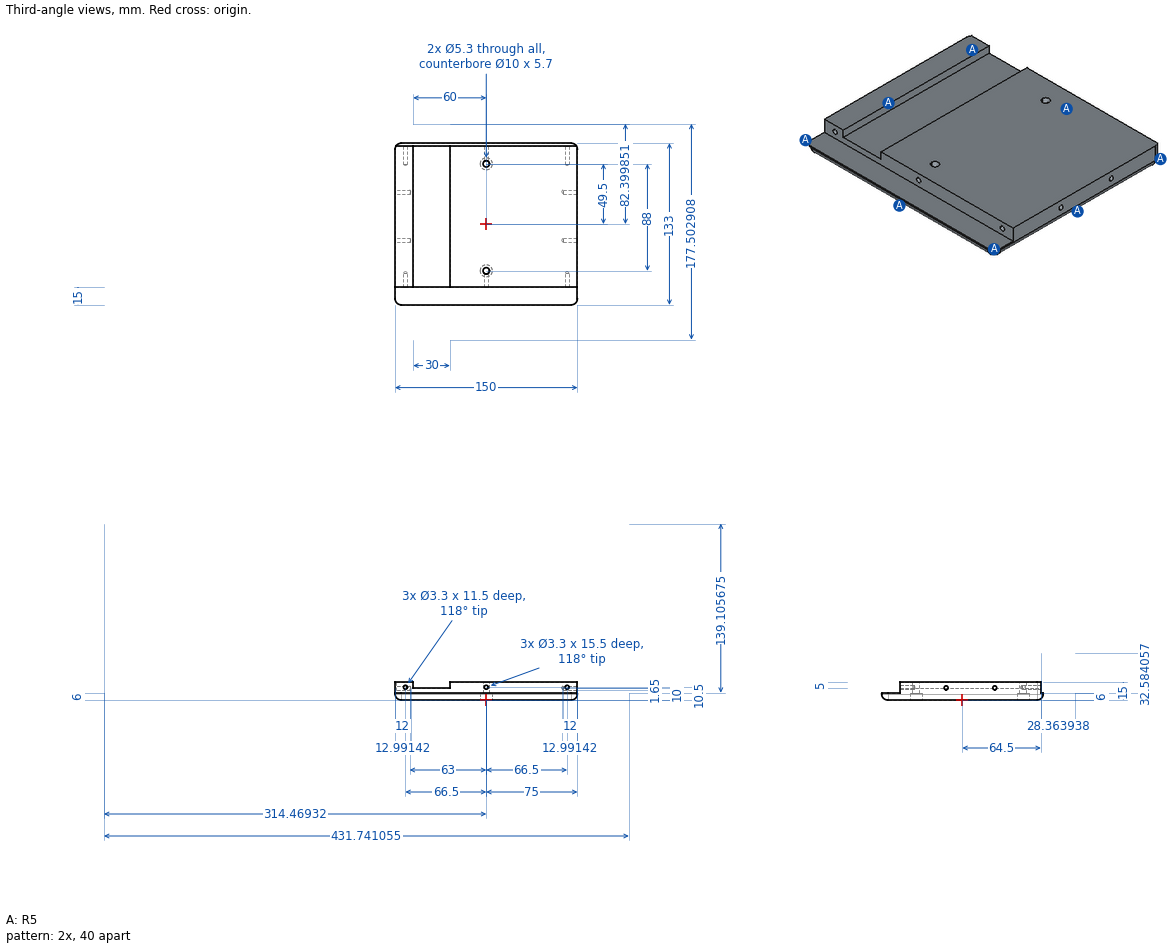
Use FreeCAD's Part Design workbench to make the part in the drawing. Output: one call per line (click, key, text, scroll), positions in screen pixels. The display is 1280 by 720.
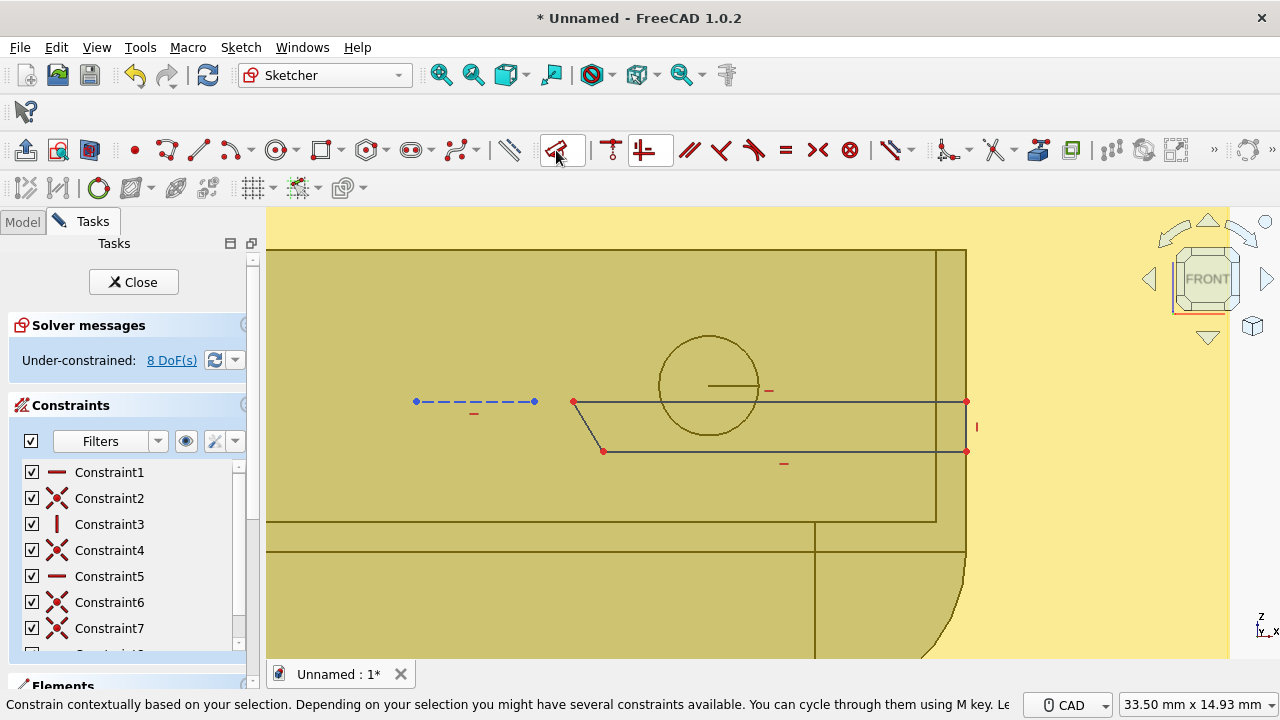
click(857, 452)
click(784, 486)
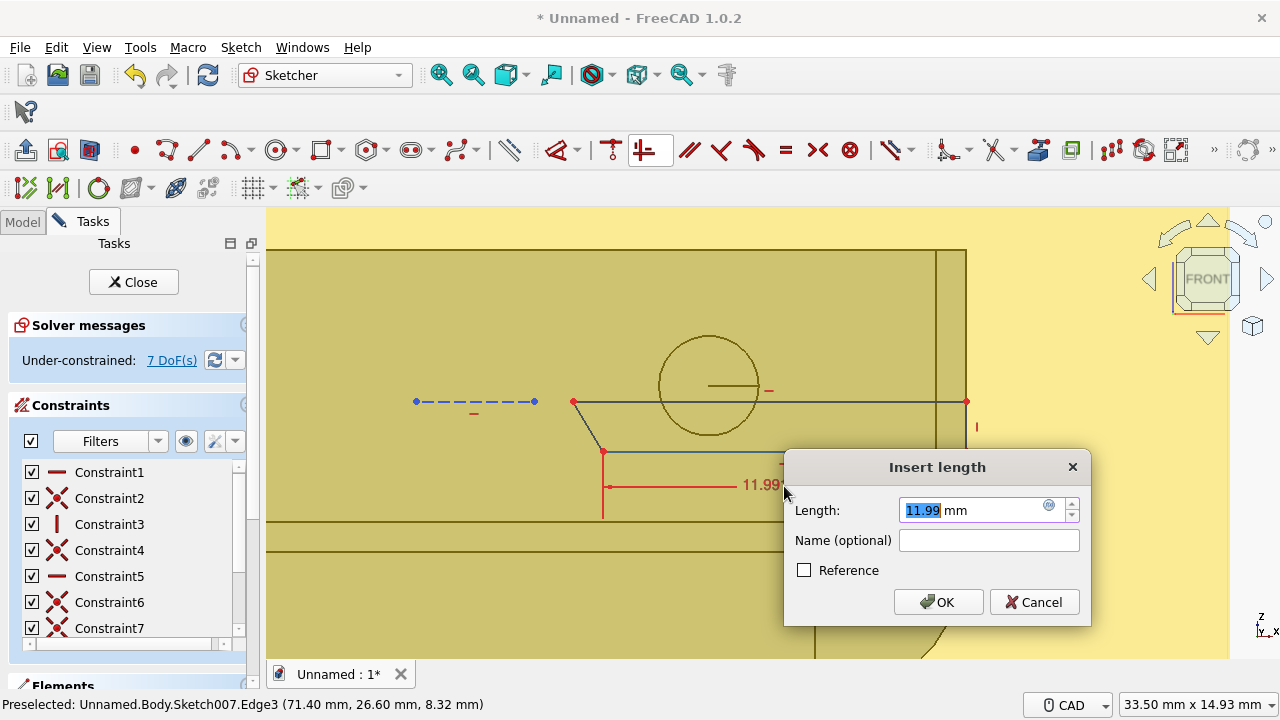
text(12)
key(Return)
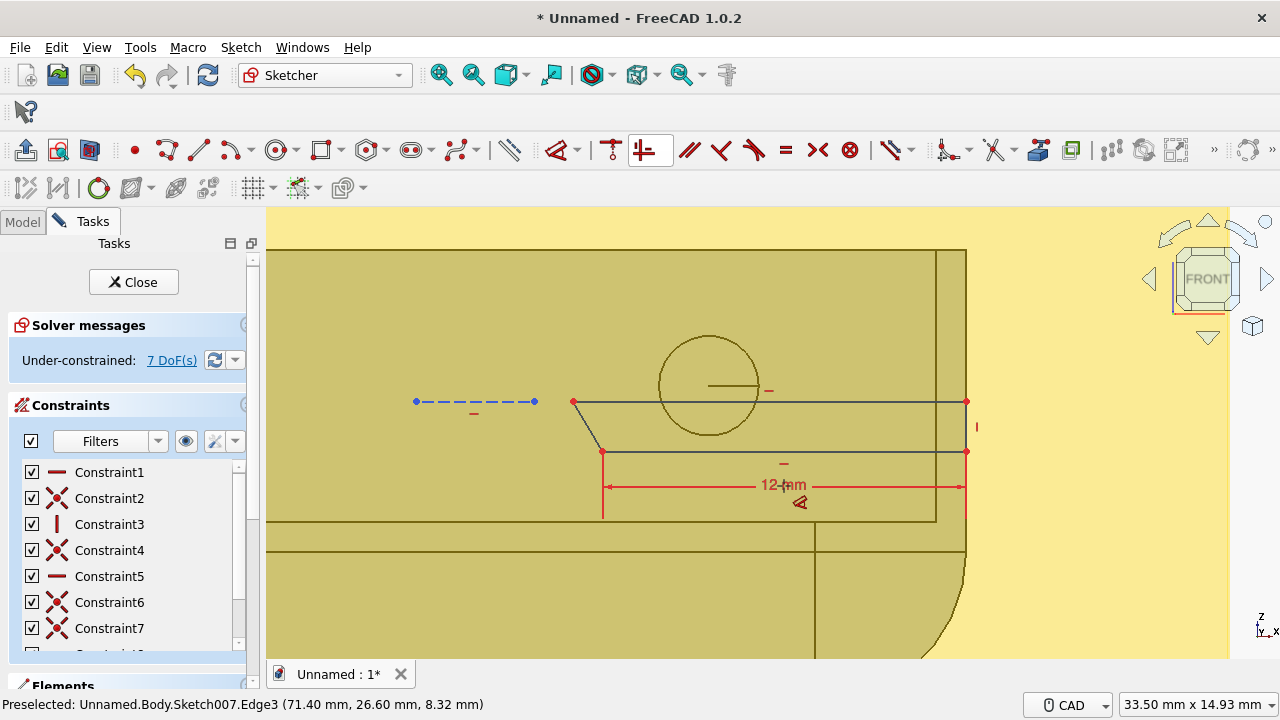
click(573, 402)
click(607, 516)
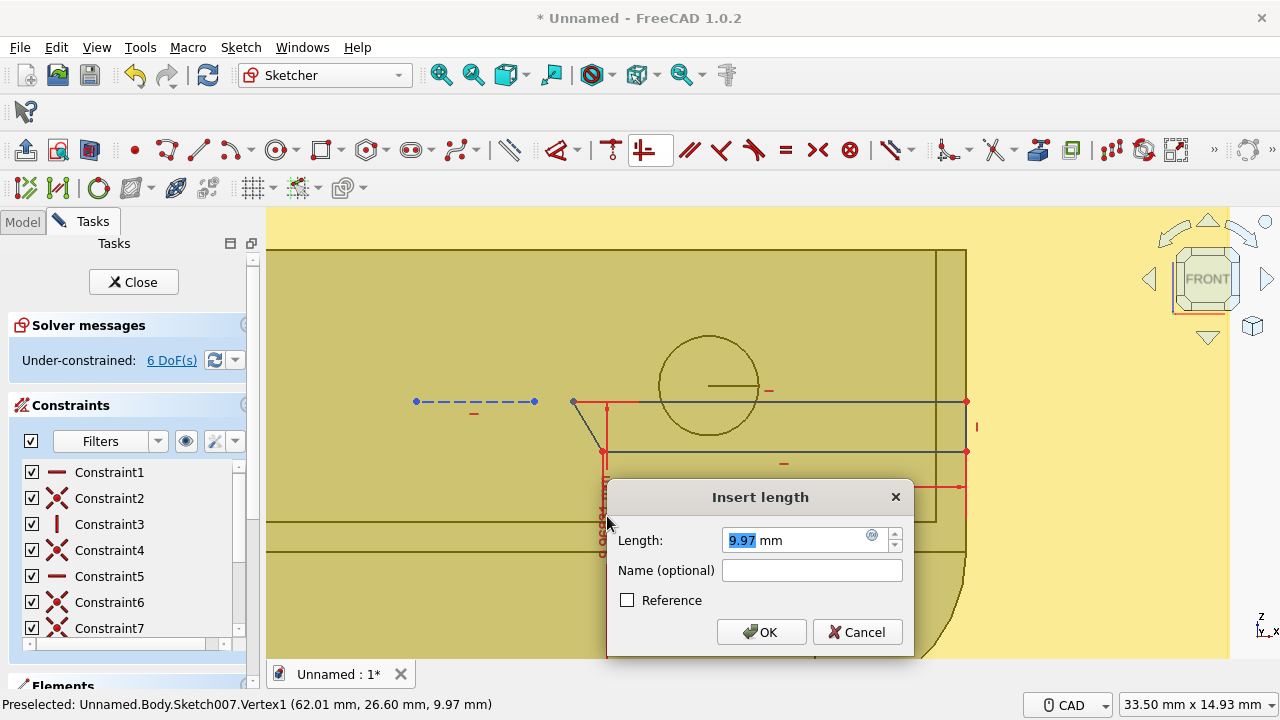
text(10)
key(Return)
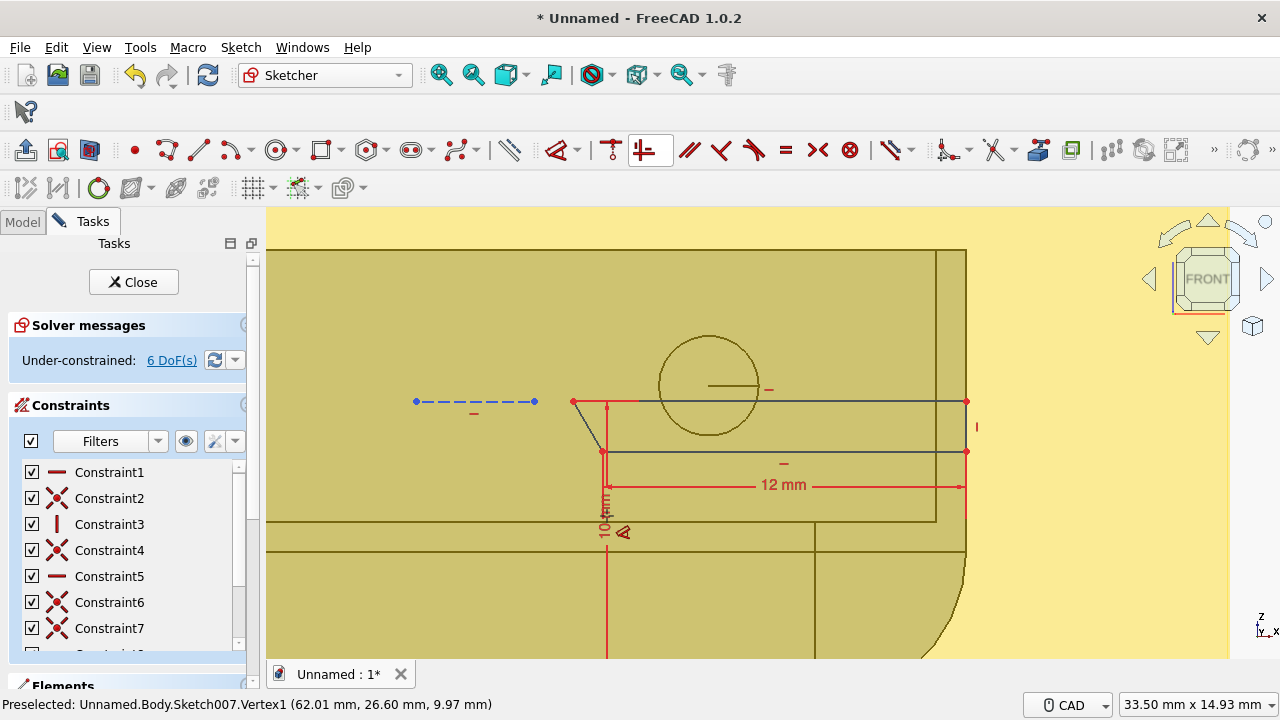
click(966, 401)
click(630, 367)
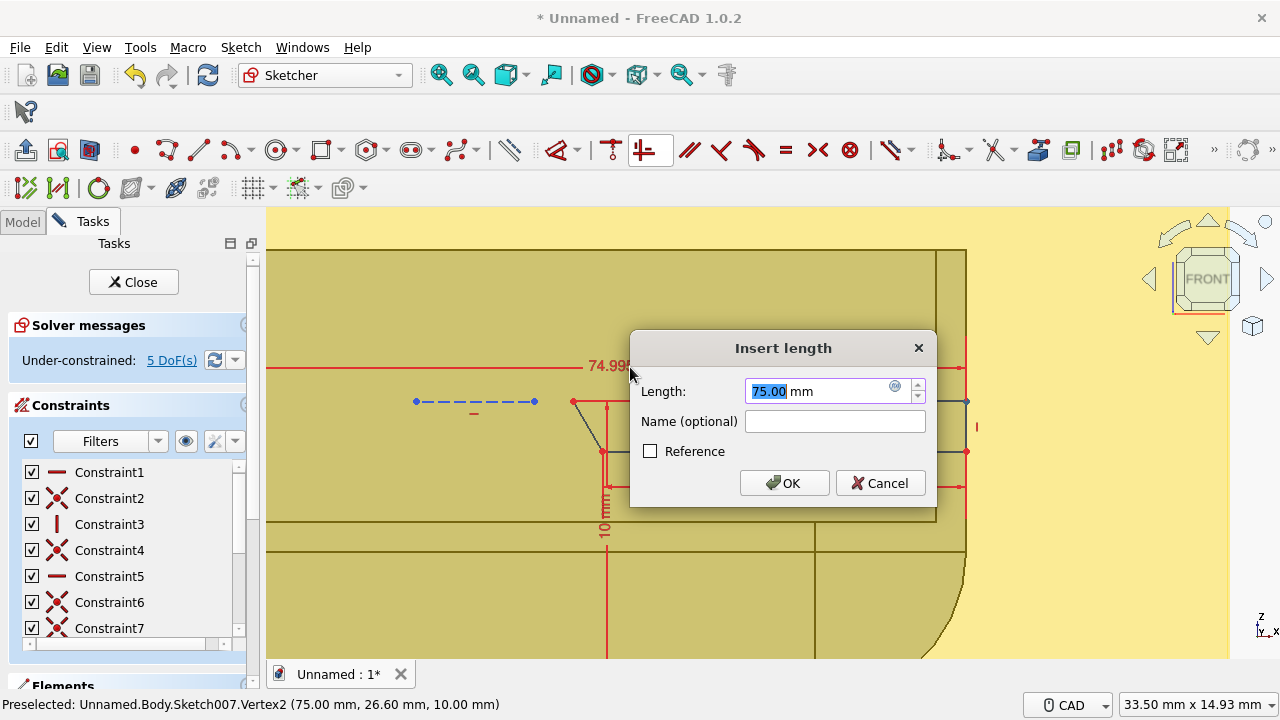
text(75)
key(Return)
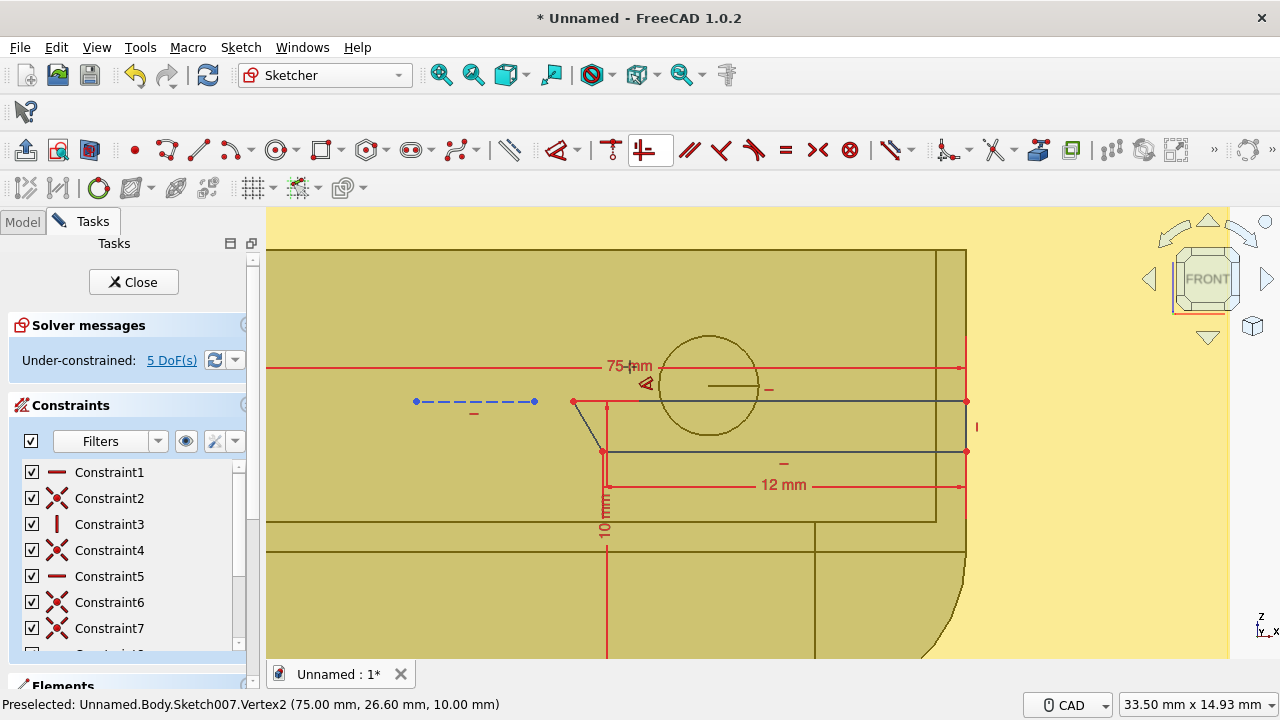
click(534, 402)
click(568, 464)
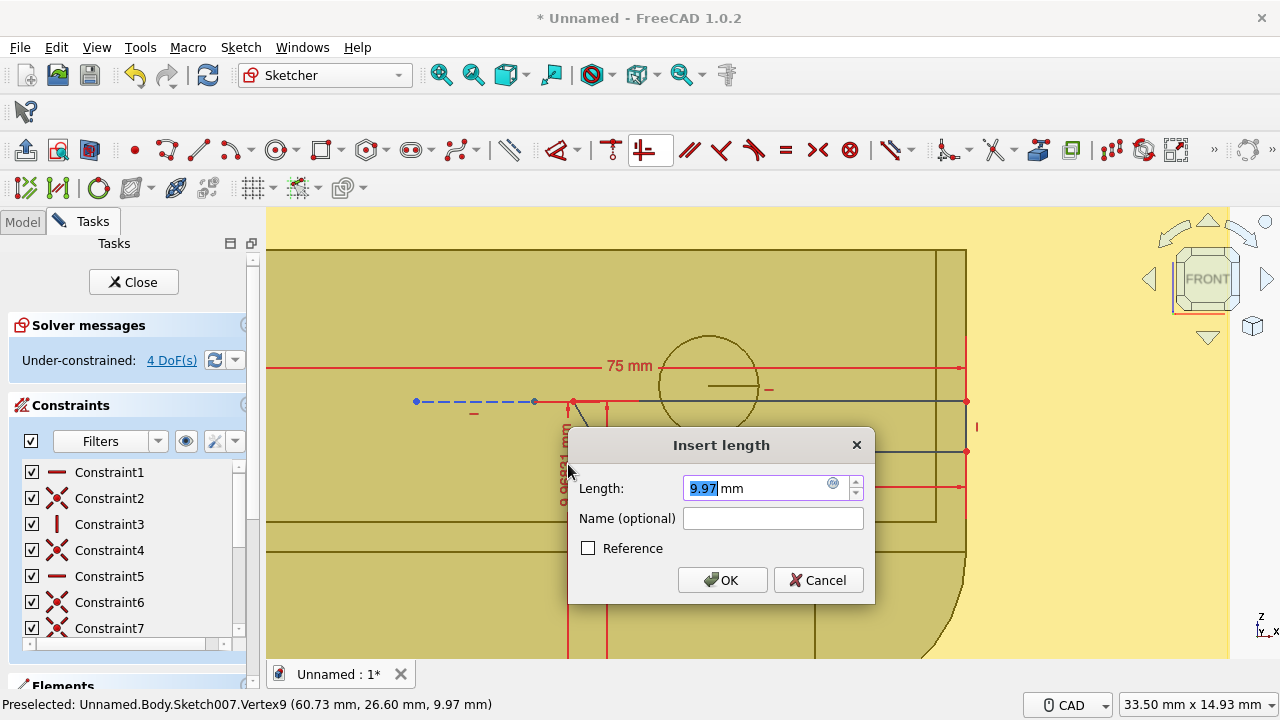
text(10)
key(Return)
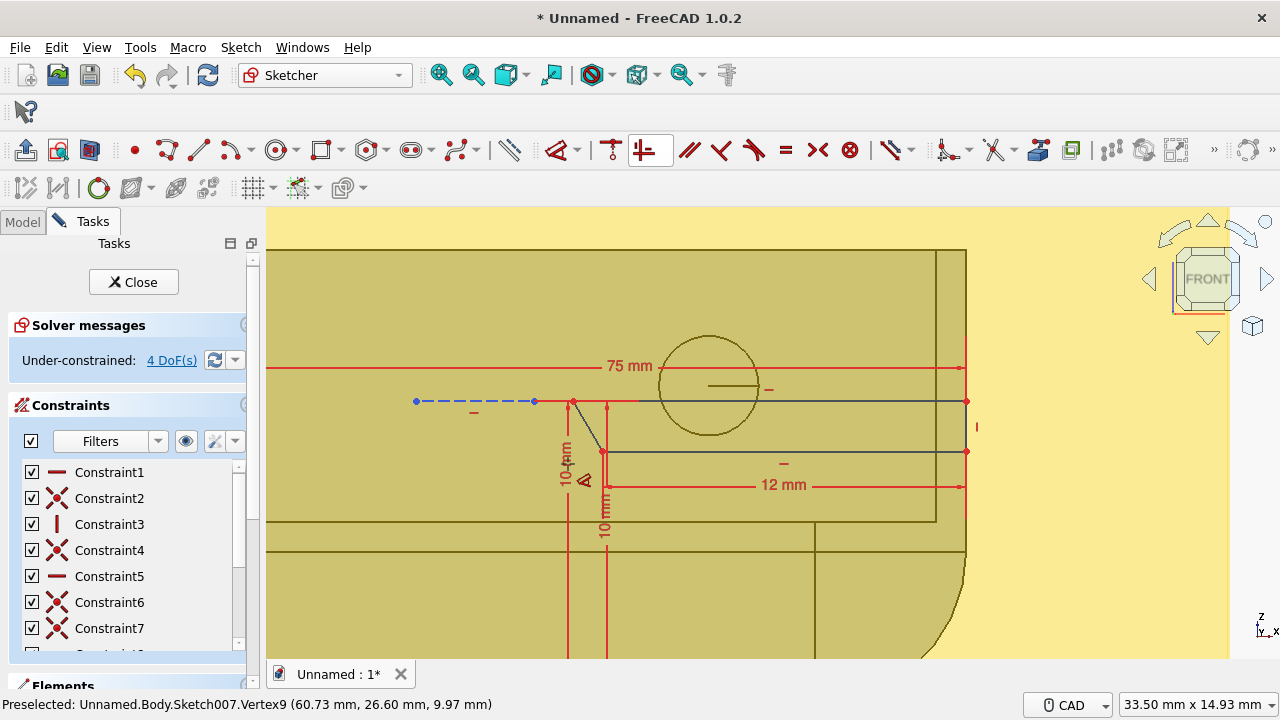
click(966, 416)
click(1000, 427)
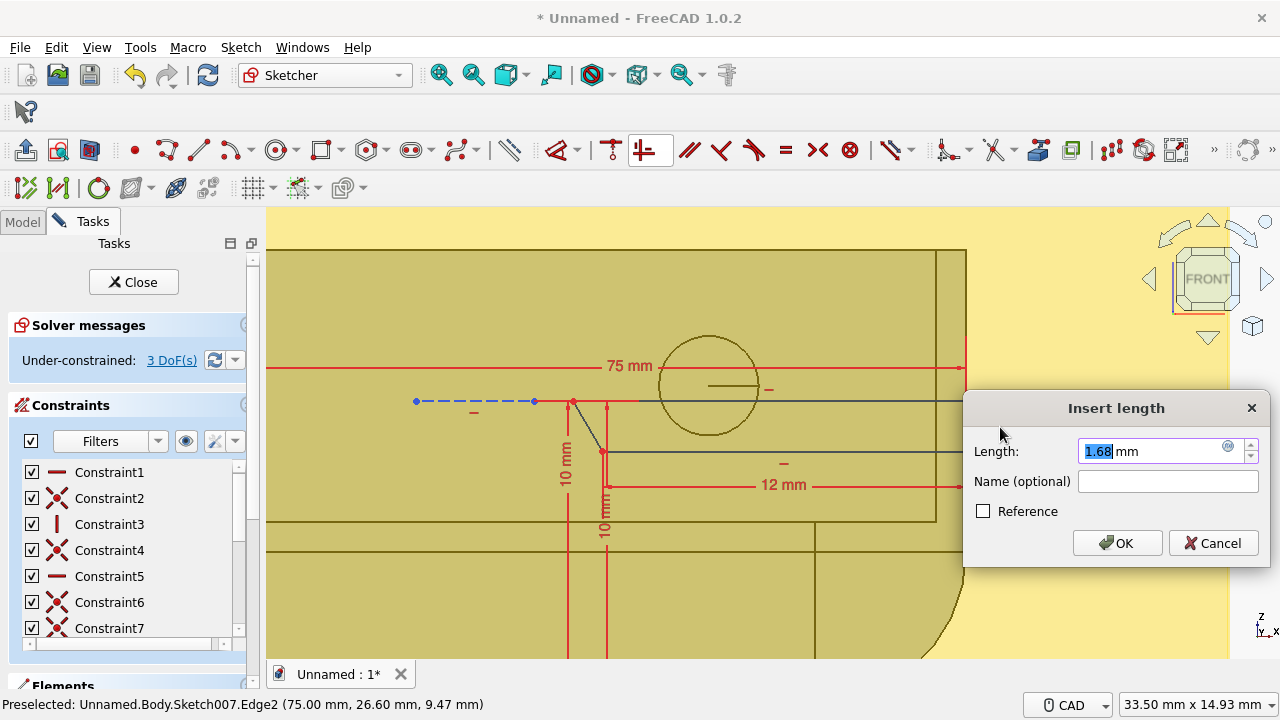
text(1.65)
key(Return)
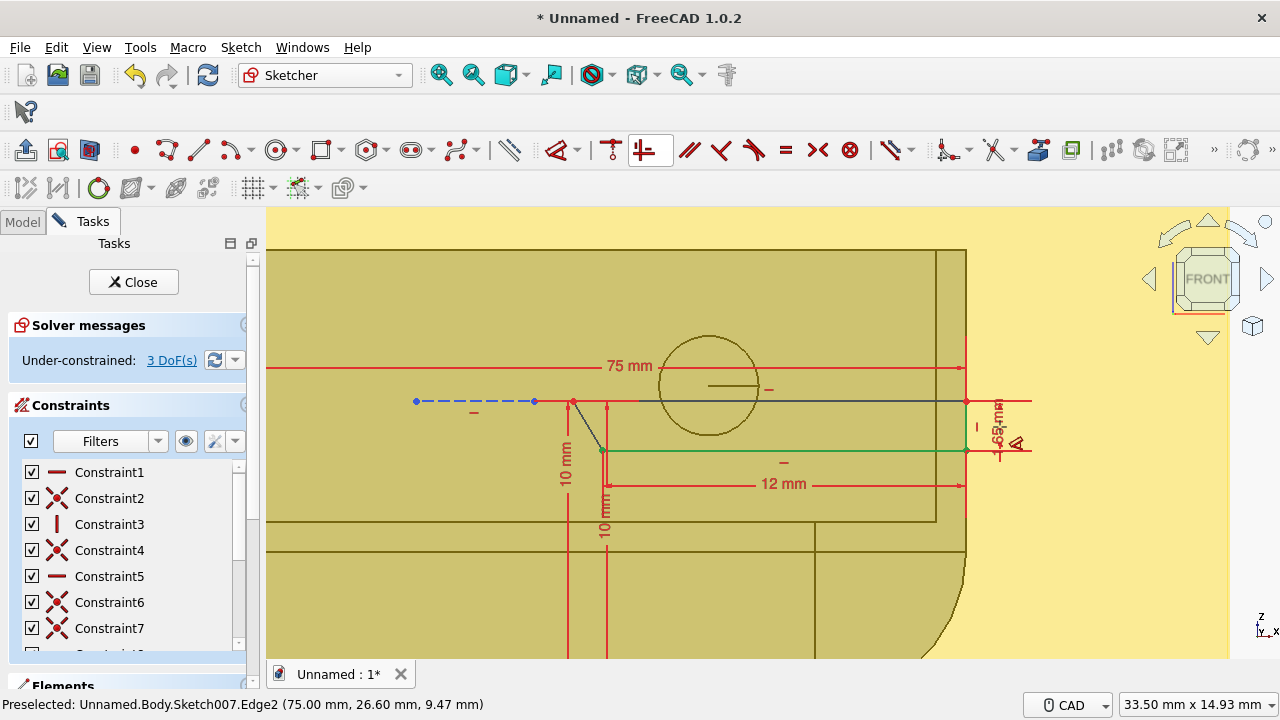
click(691, 401)
click(770, 367)